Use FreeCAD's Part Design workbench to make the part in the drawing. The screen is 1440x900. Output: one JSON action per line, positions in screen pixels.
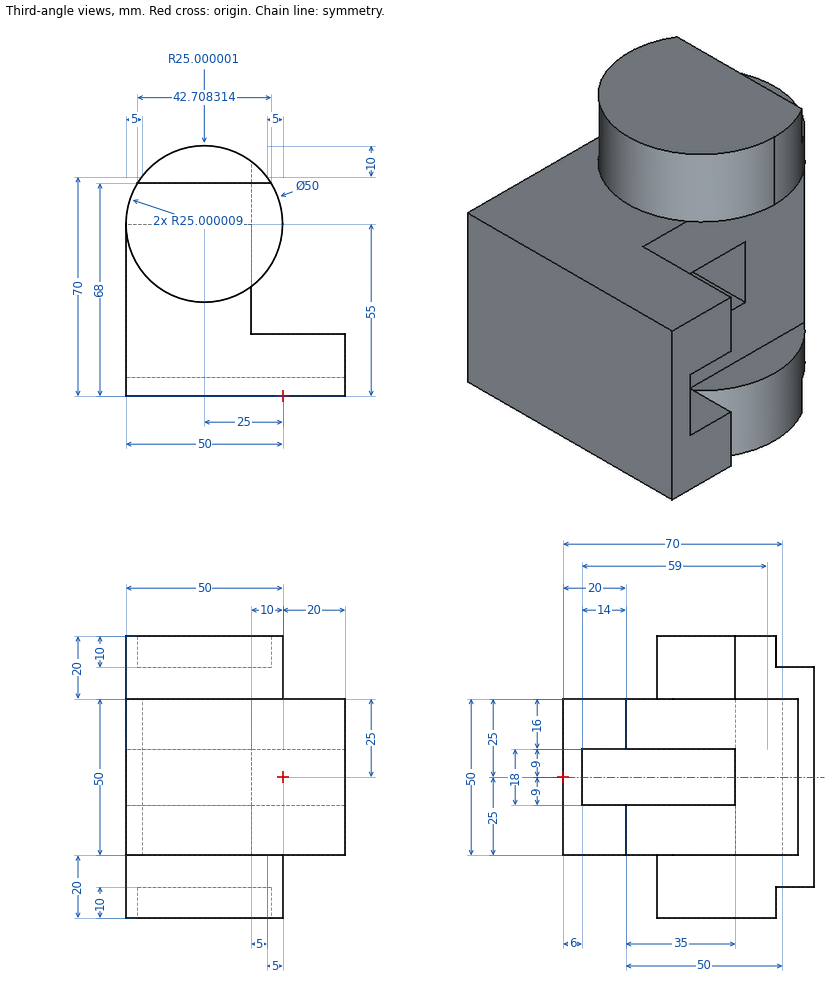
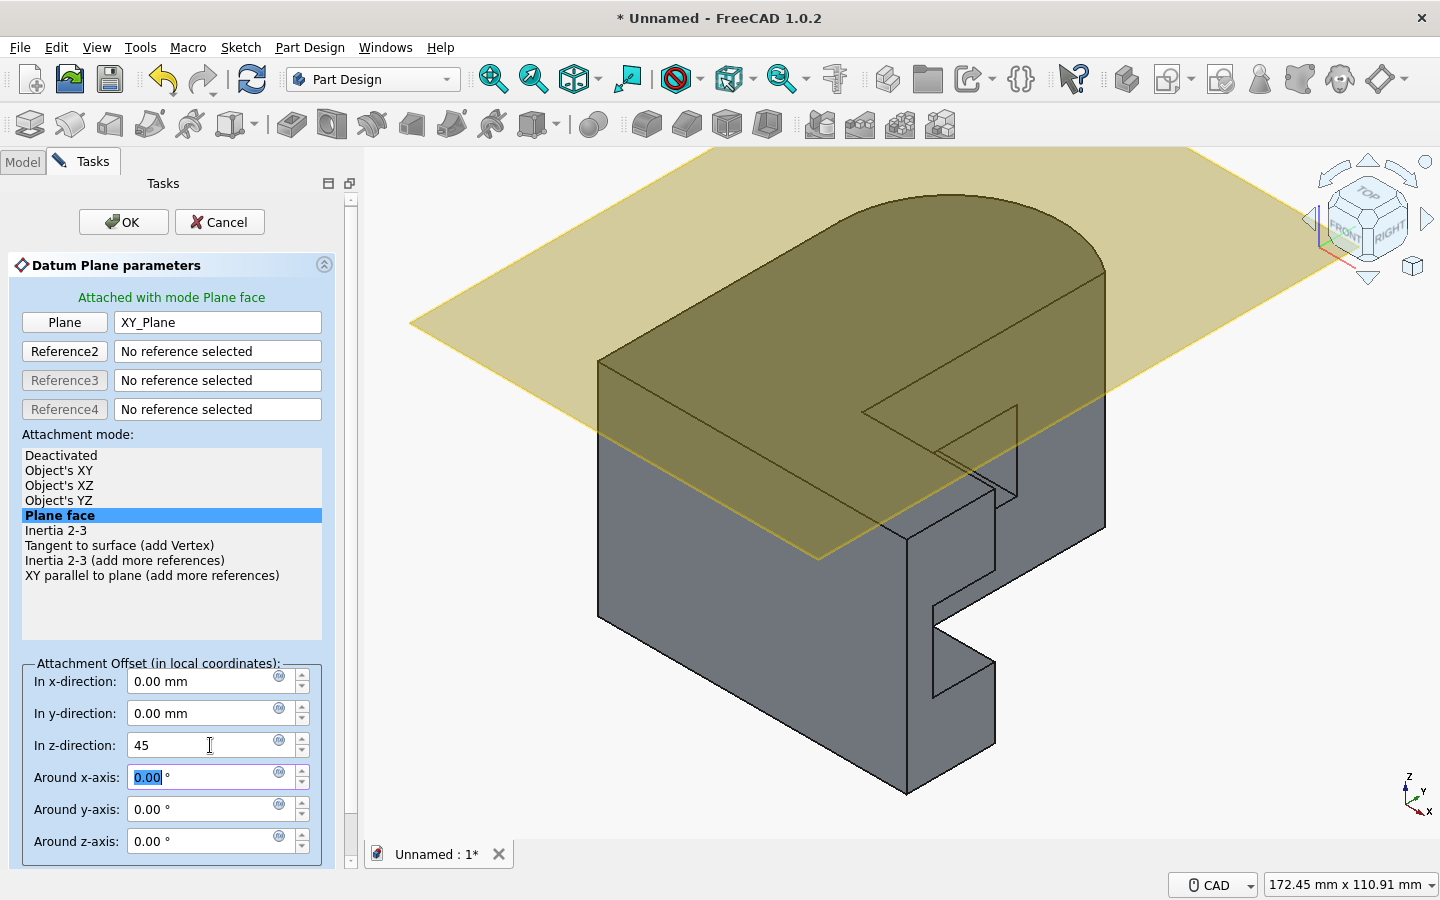
{"action": "left_click", "coordinate": [124, 222]}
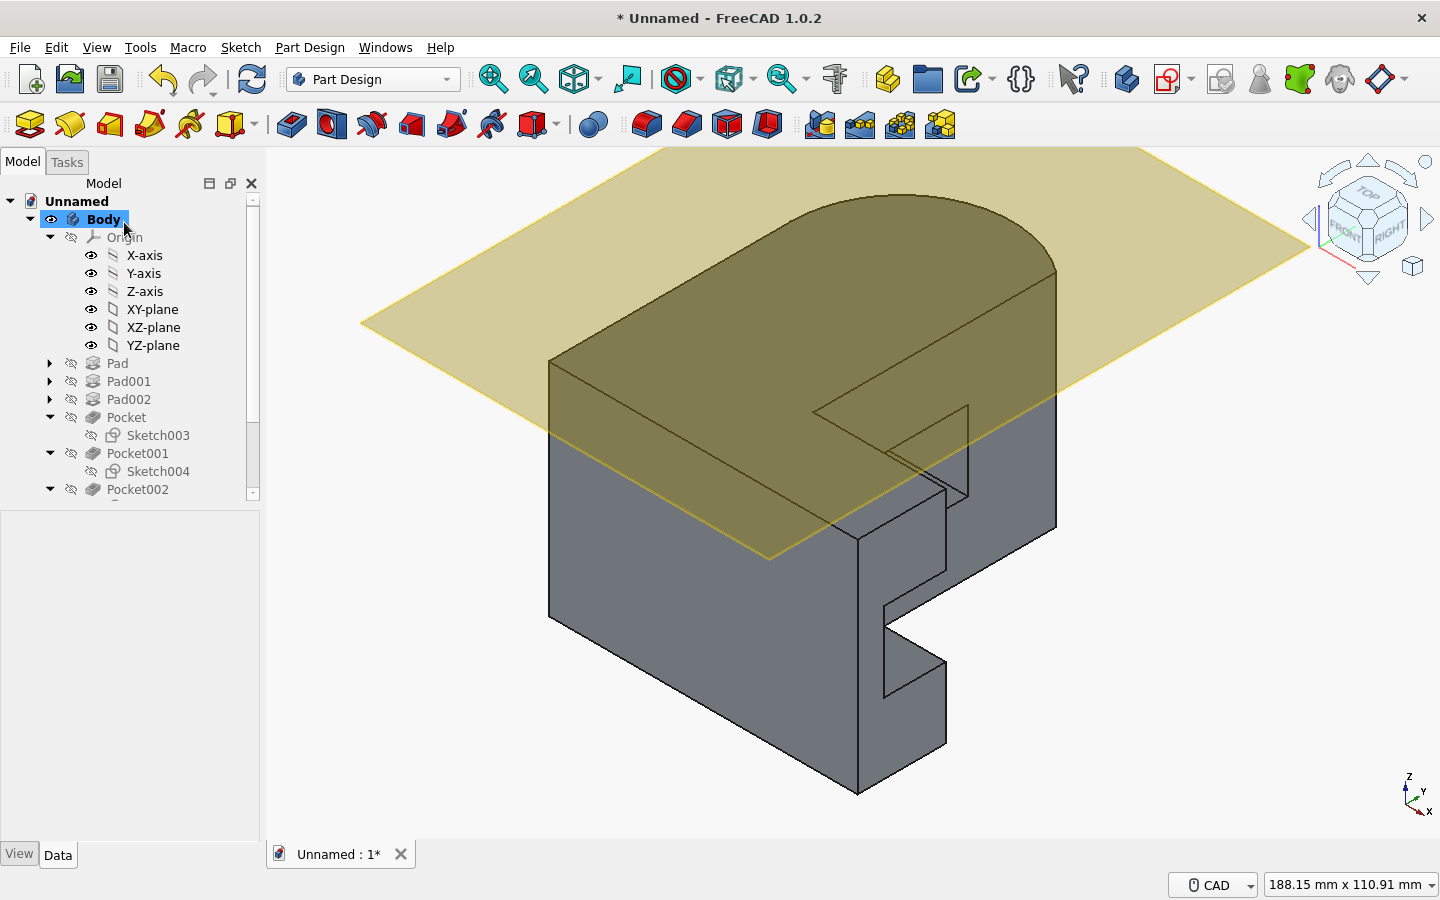
{"action": "scroll", "coordinate": [100, 341], "scroll_direction": "down", "scroll_amount": 3}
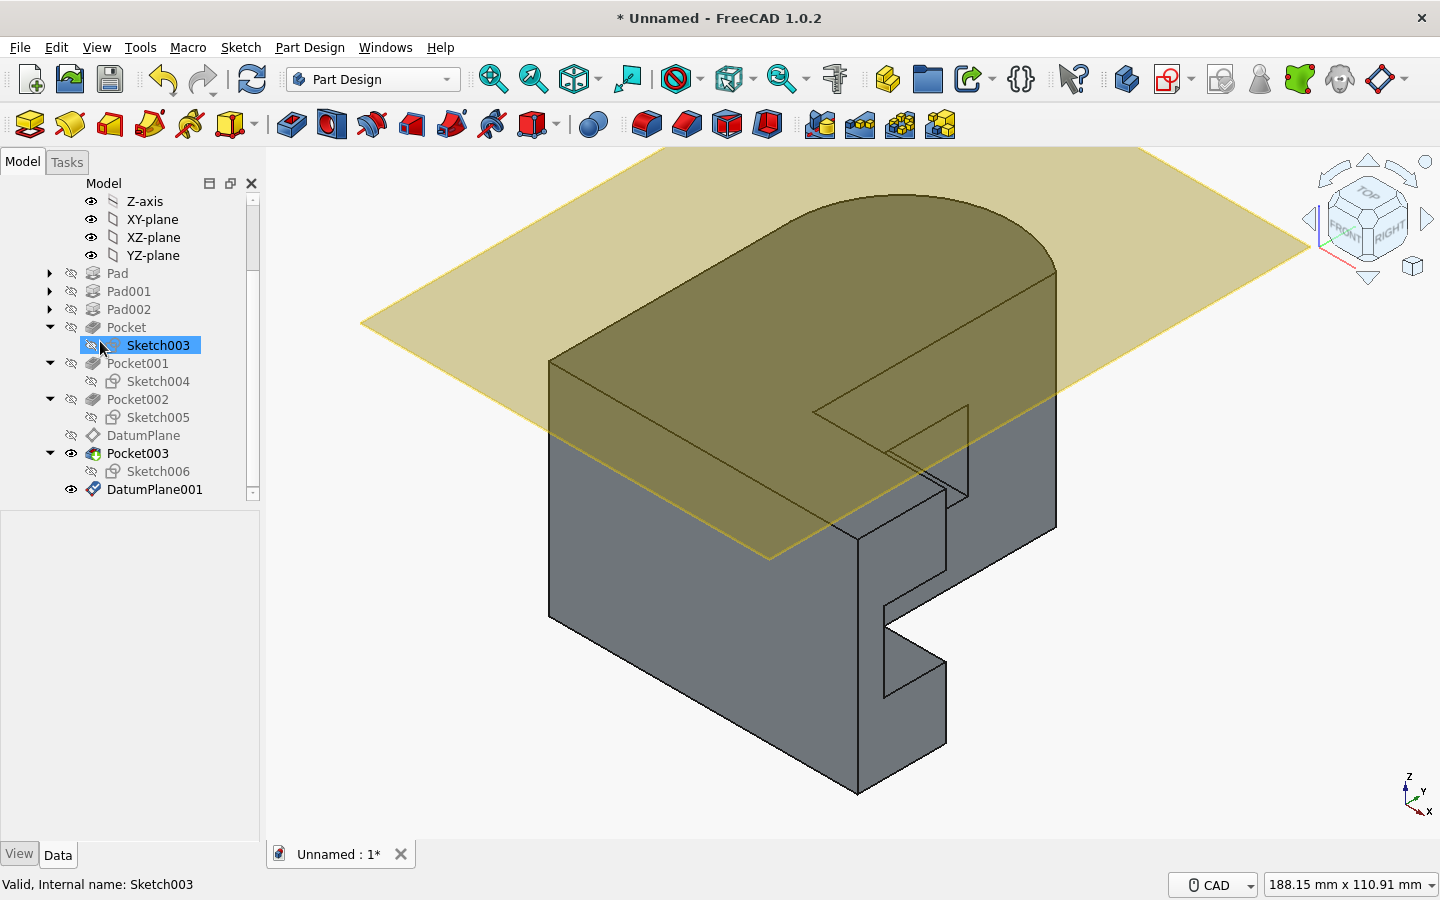
{"action": "left_click", "coordinate": [116, 489]}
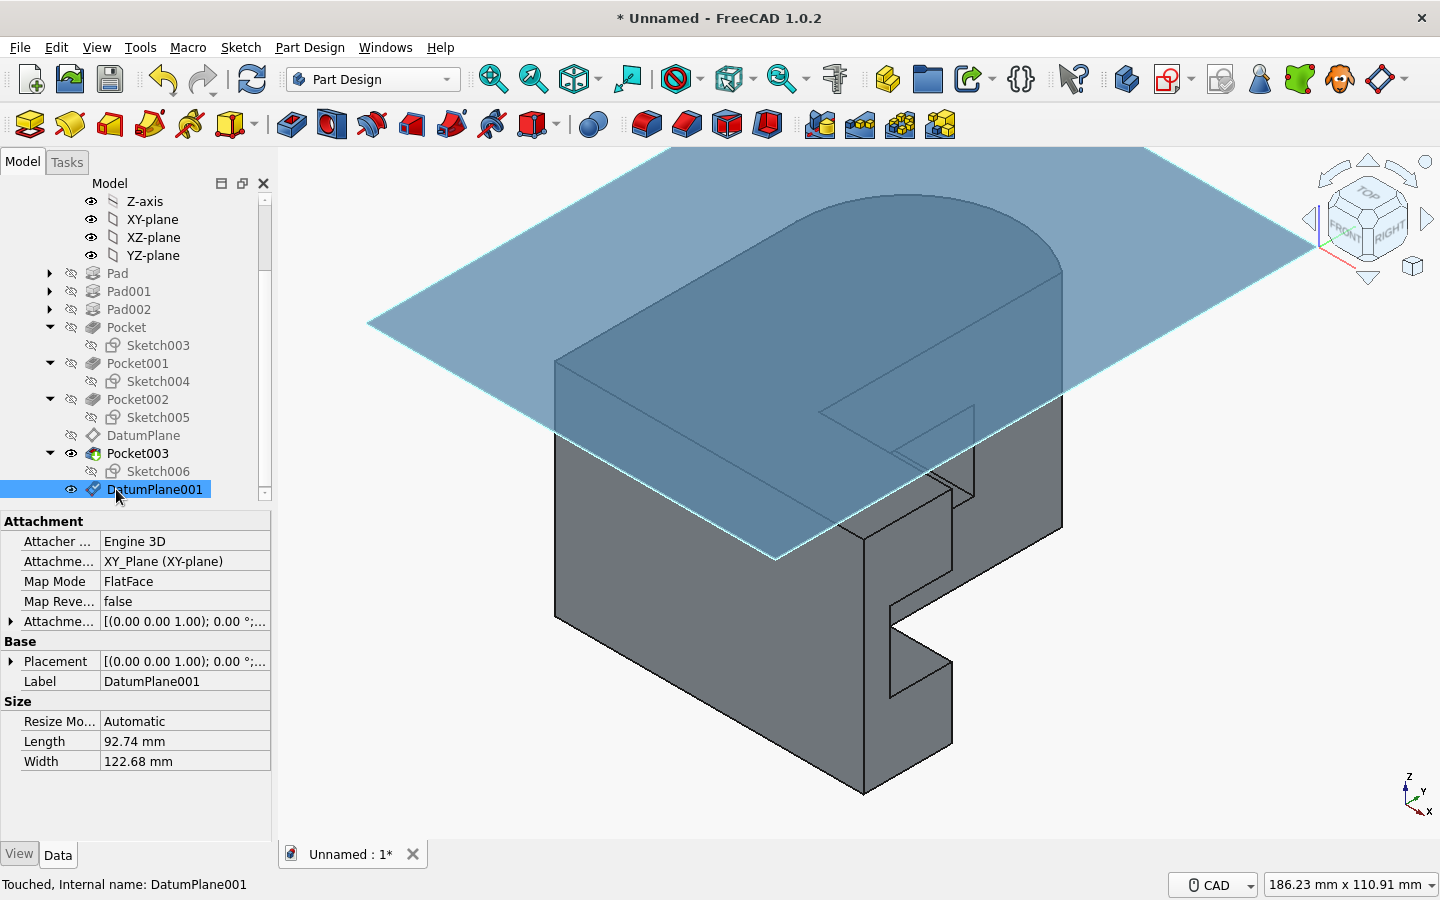
{"action": "left_click", "coordinate": [1168, 80]}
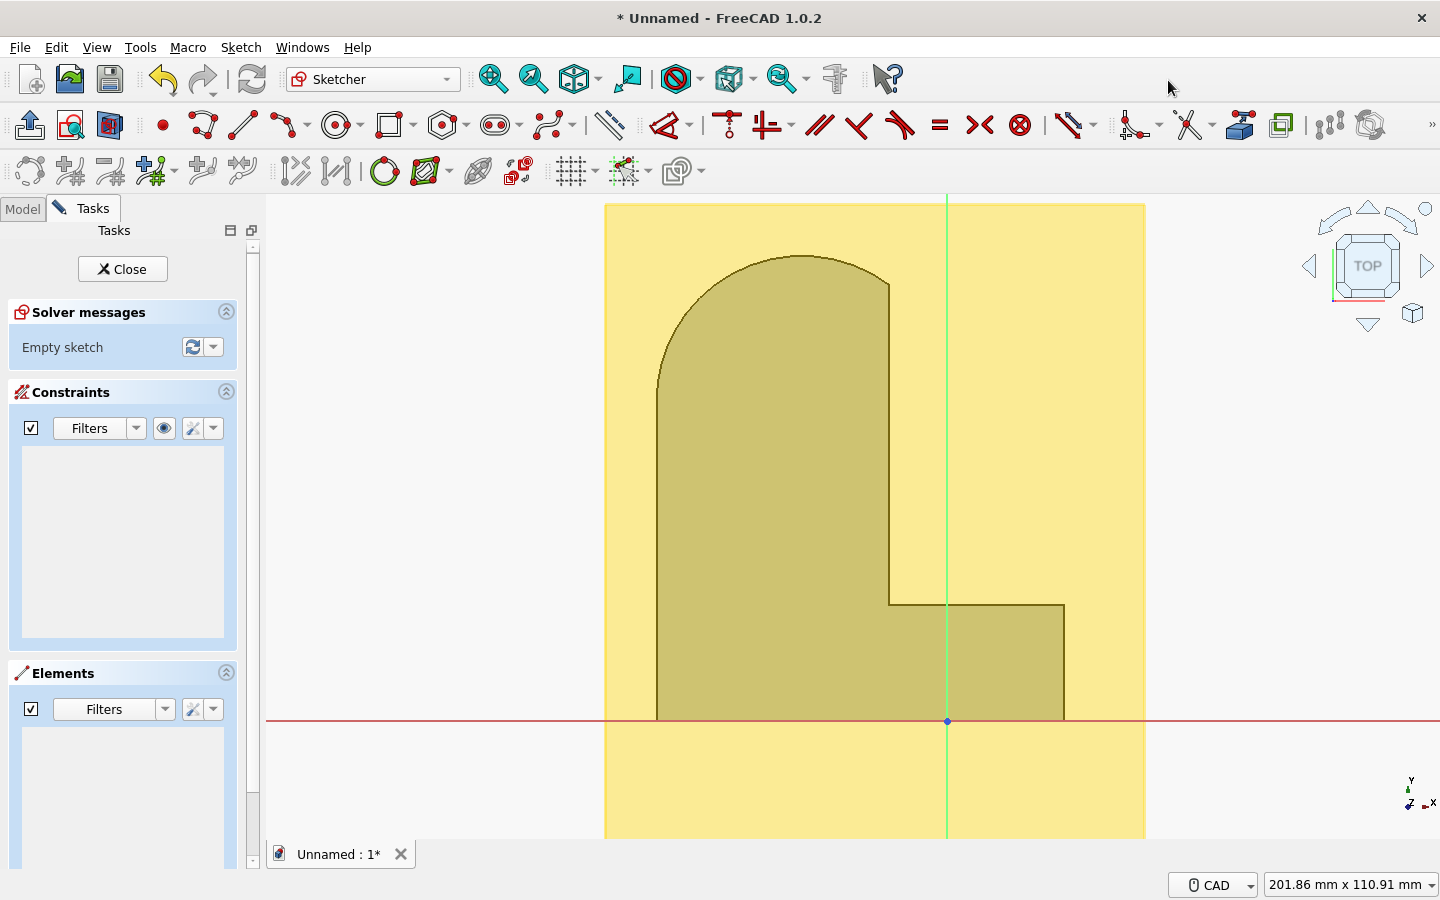
{"action": "key", "text": "g c"}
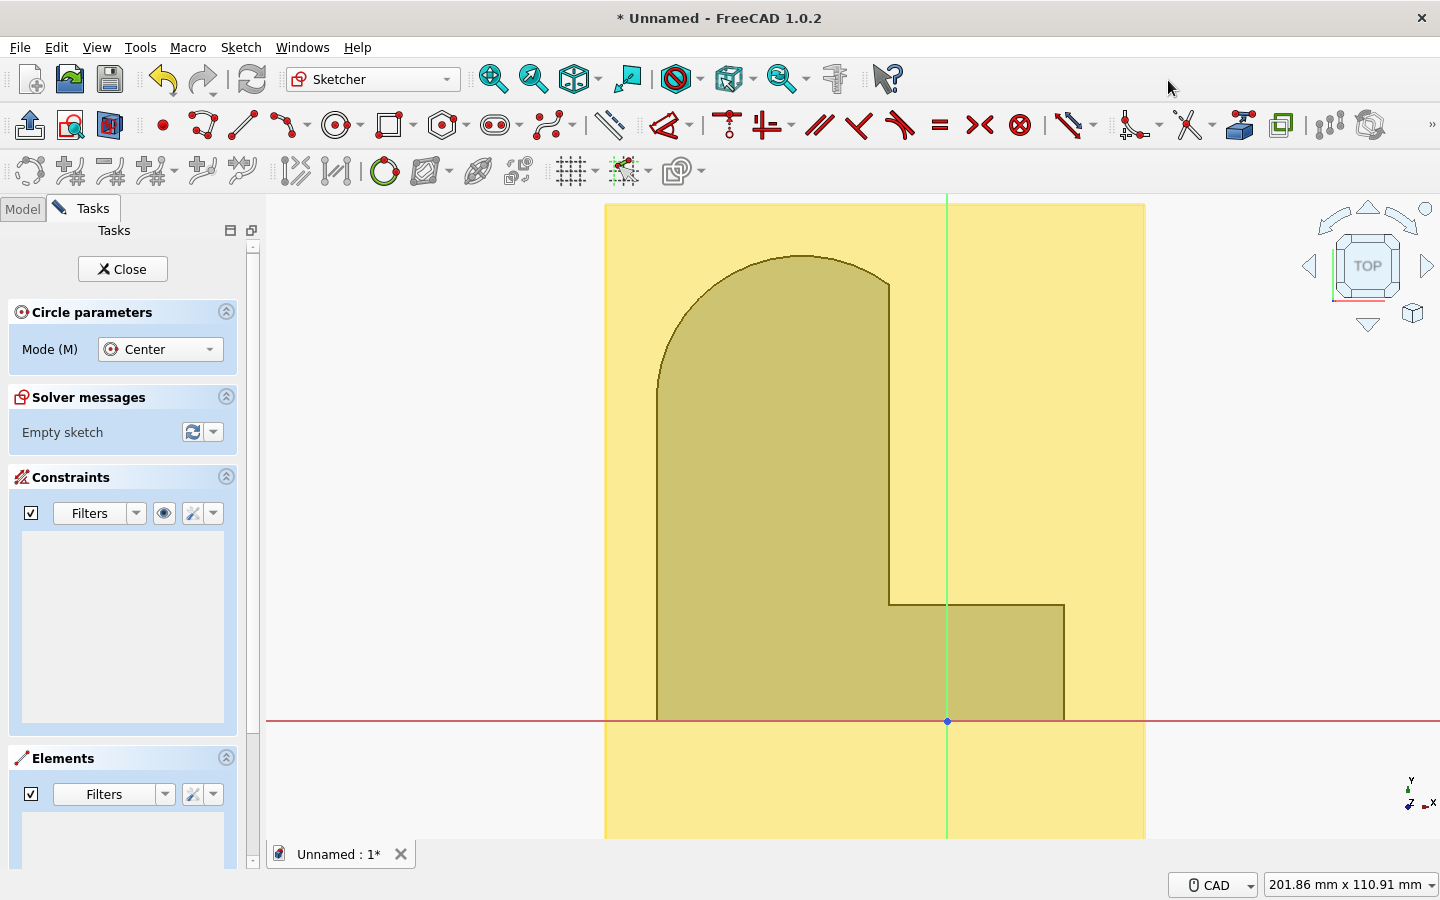
{"action": "left_click", "coordinate": [802, 401]}
{"action": "mouse_move", "coordinate": [905, 298]}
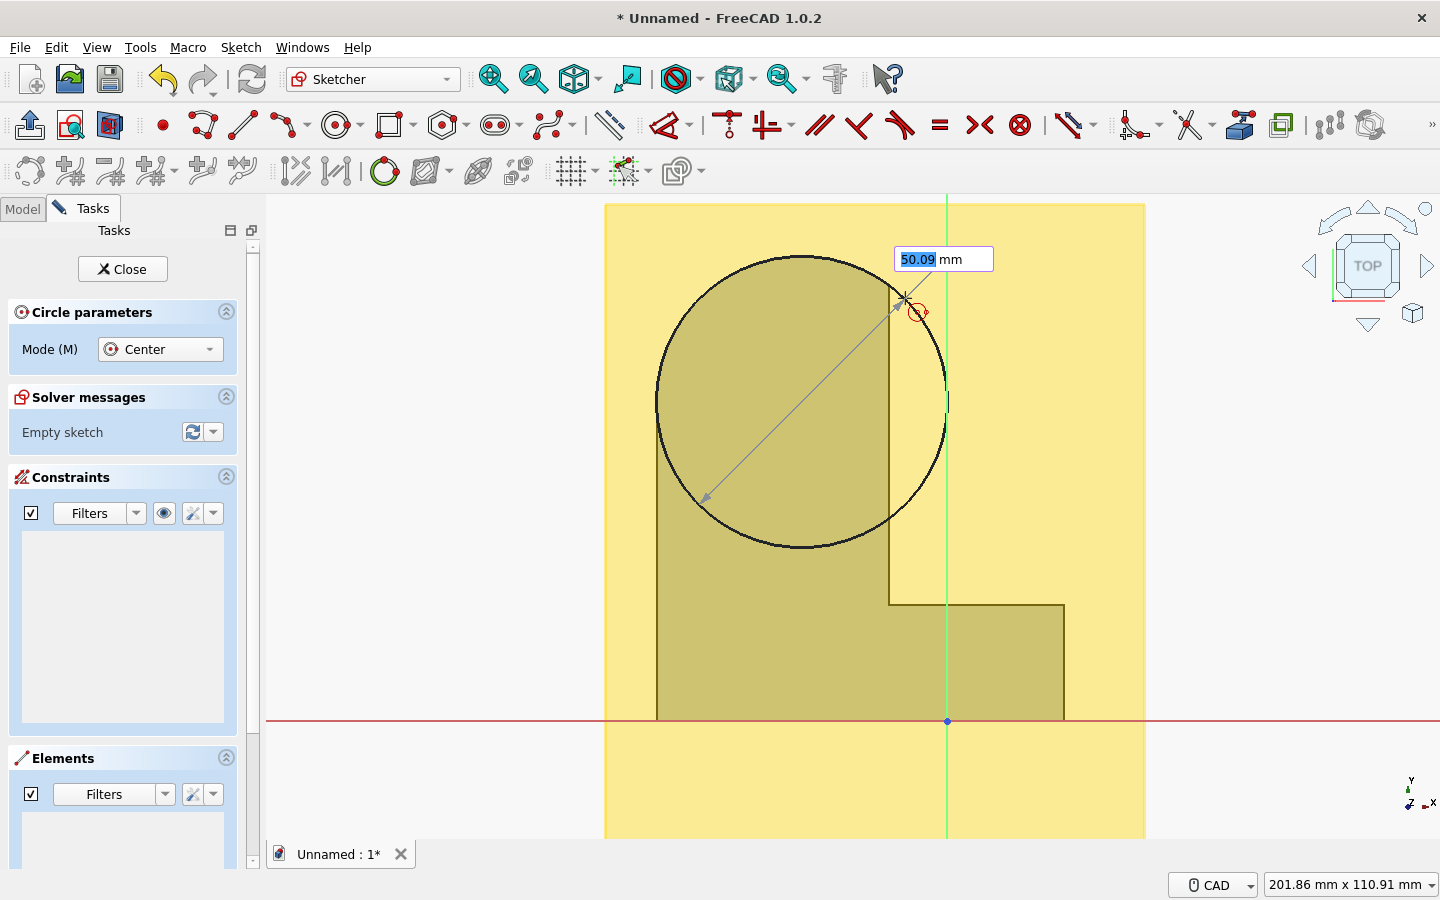
{"action": "type", "text": "50"}
{"action": "key", "text": "Return"}
{"action": "key", "text": "Escape"}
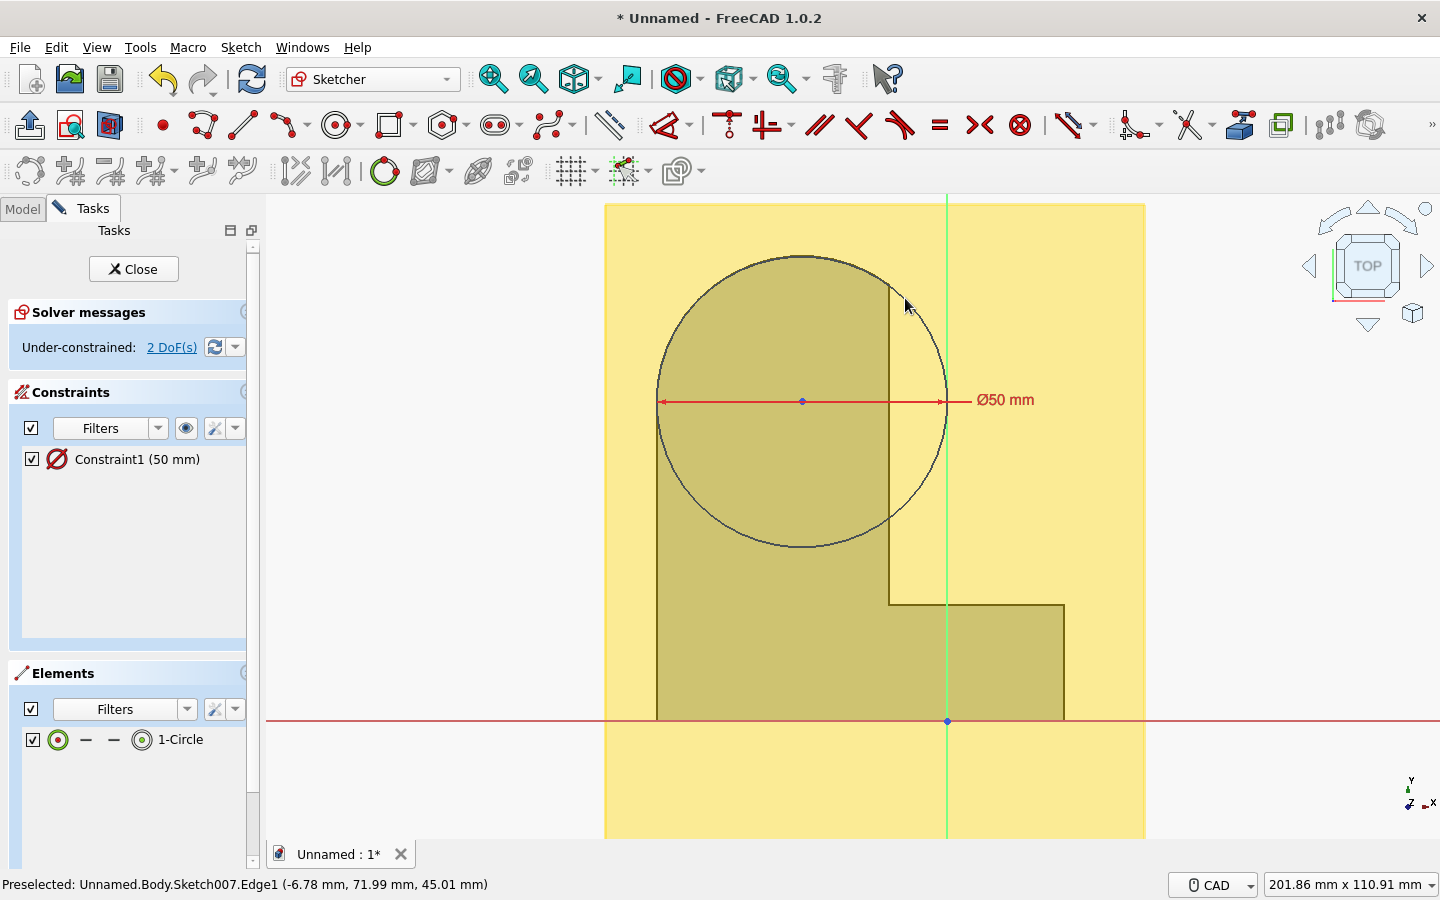
{"action": "left_click", "coordinate": [664, 126]}